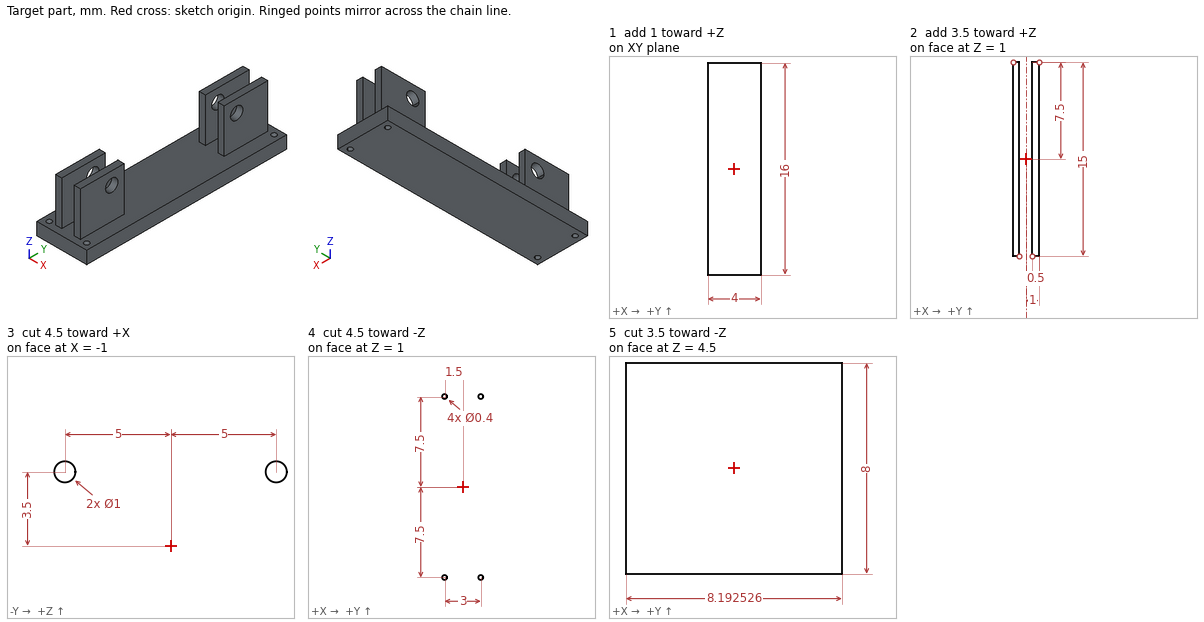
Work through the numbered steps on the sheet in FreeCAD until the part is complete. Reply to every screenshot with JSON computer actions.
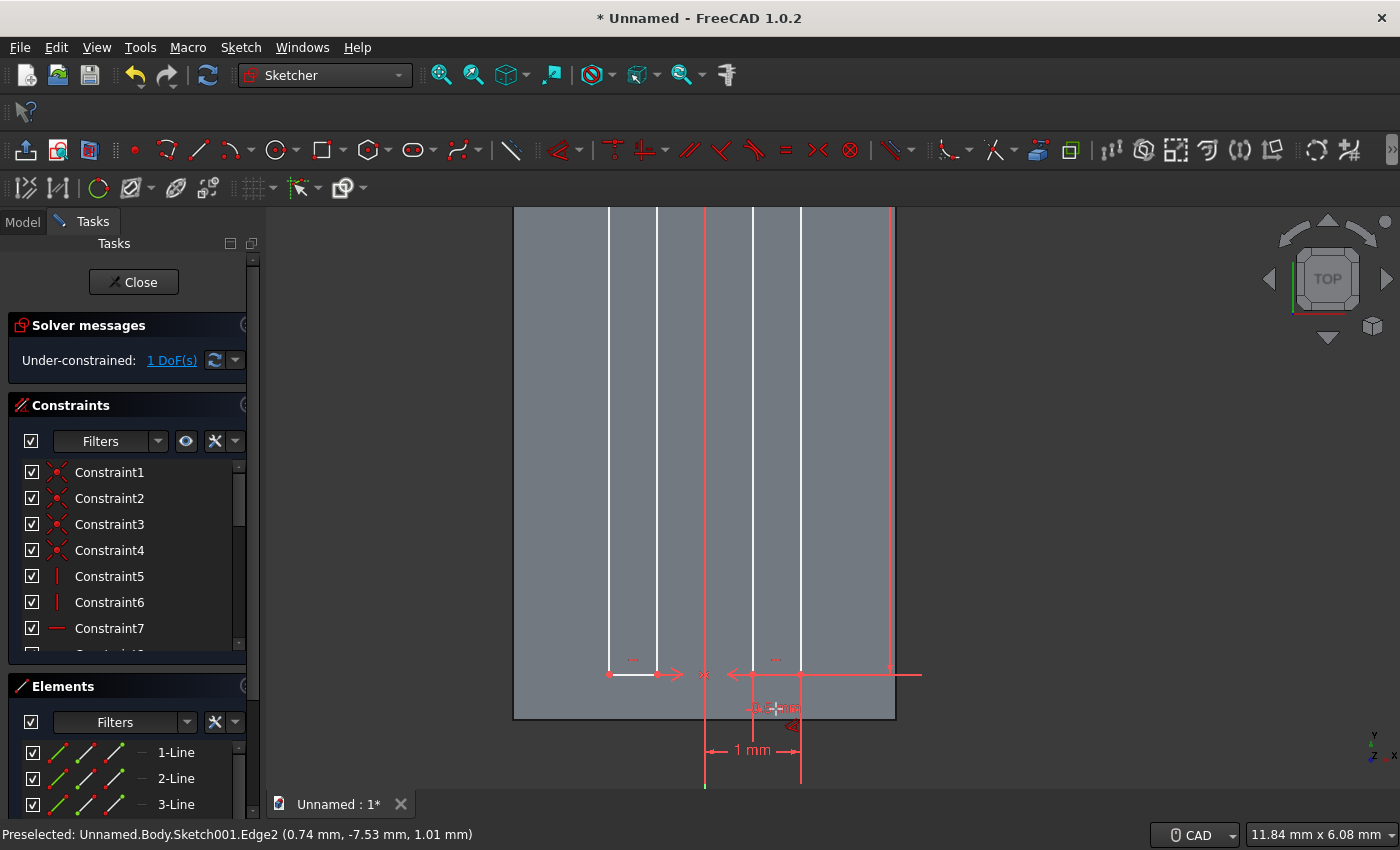
{"action": "scroll", "coordinate": [784, 676], "scroll_direction": "down", "scroll_amount": 7}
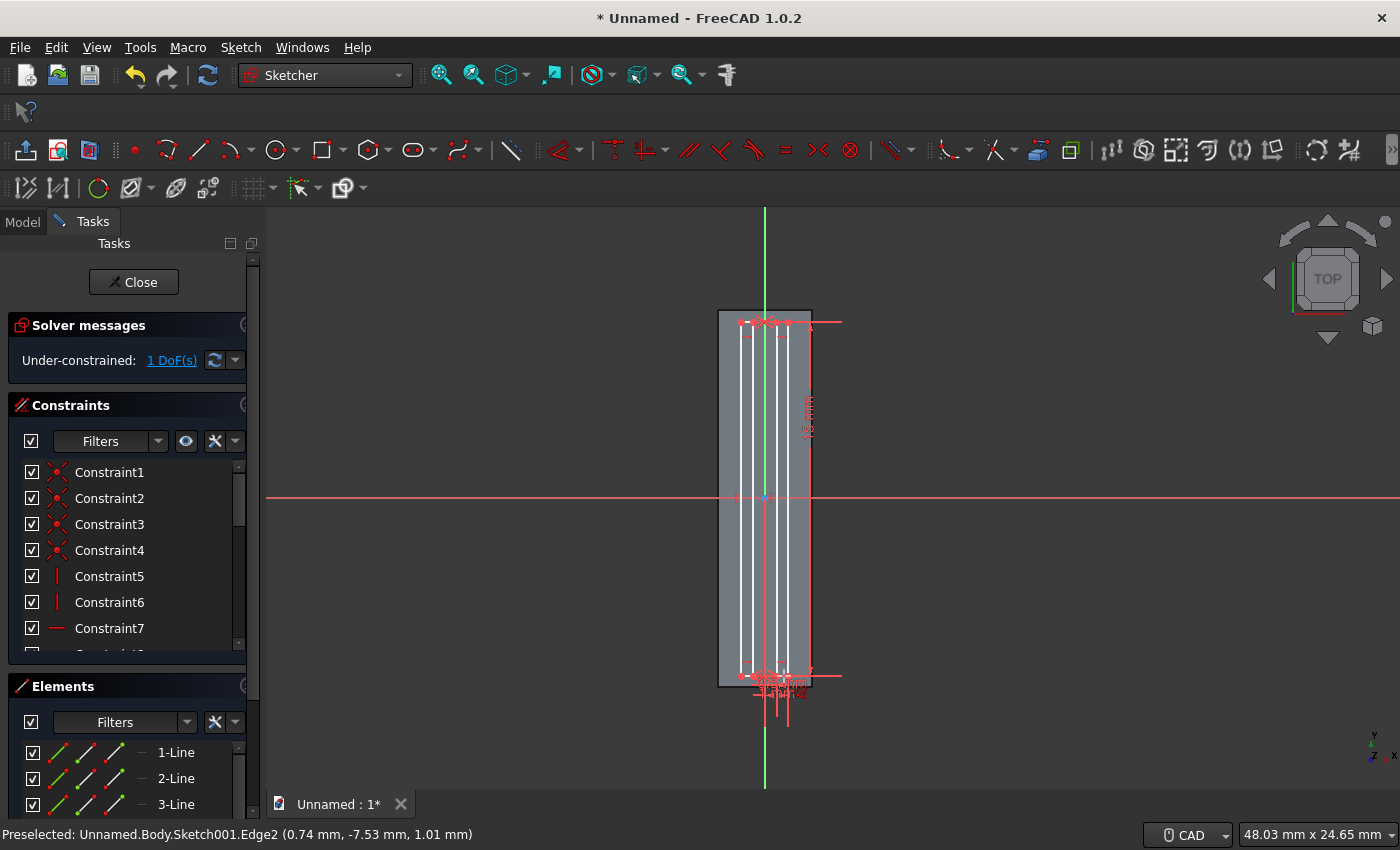
{"action": "left_click", "coordinate": [777, 322]}
{"action": "left_click", "coordinate": [811, 370]}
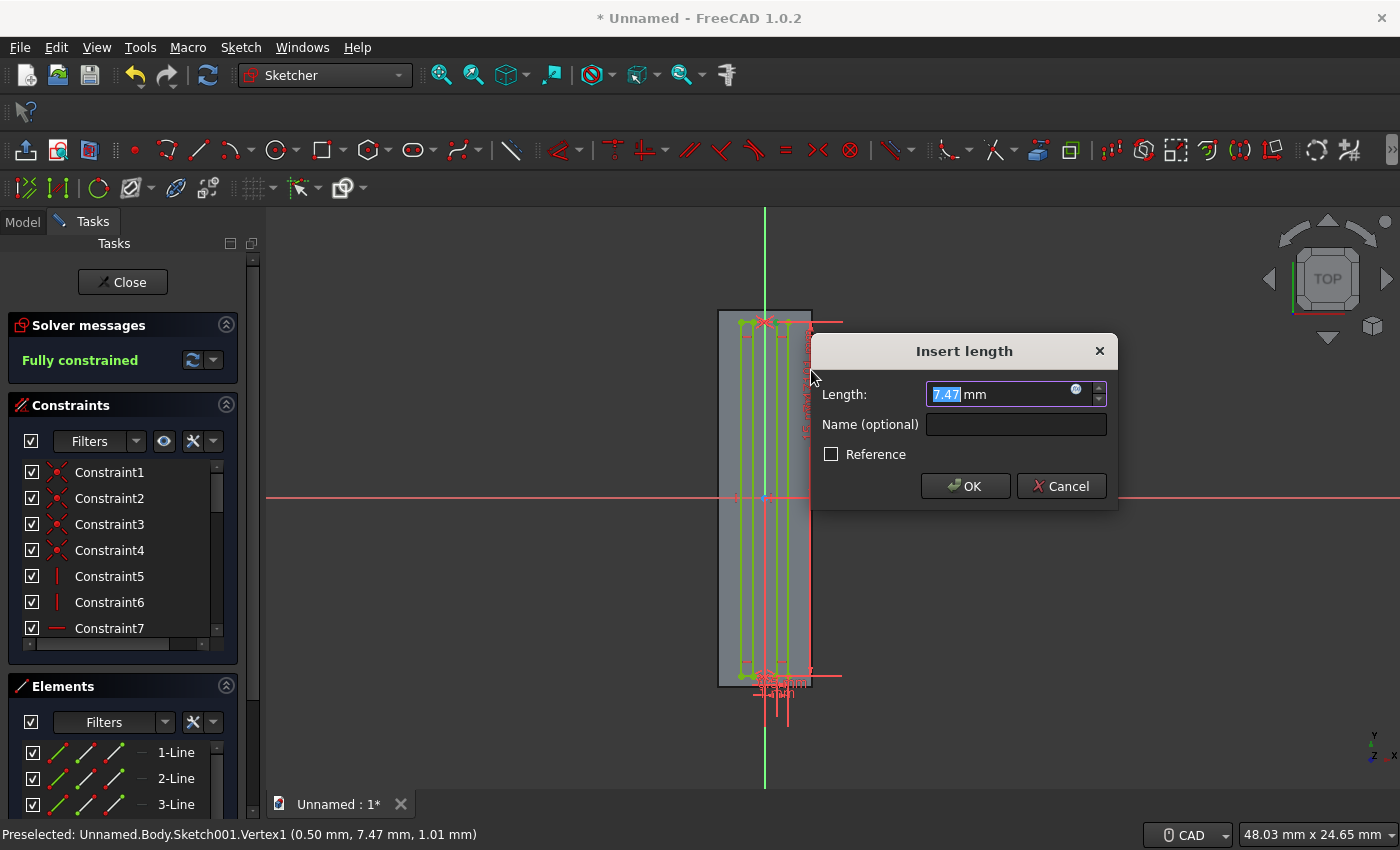
{"action": "type", "text": "7.5"}
{"action": "key", "text": "Return"}
{"action": "key", "text": "Escape"}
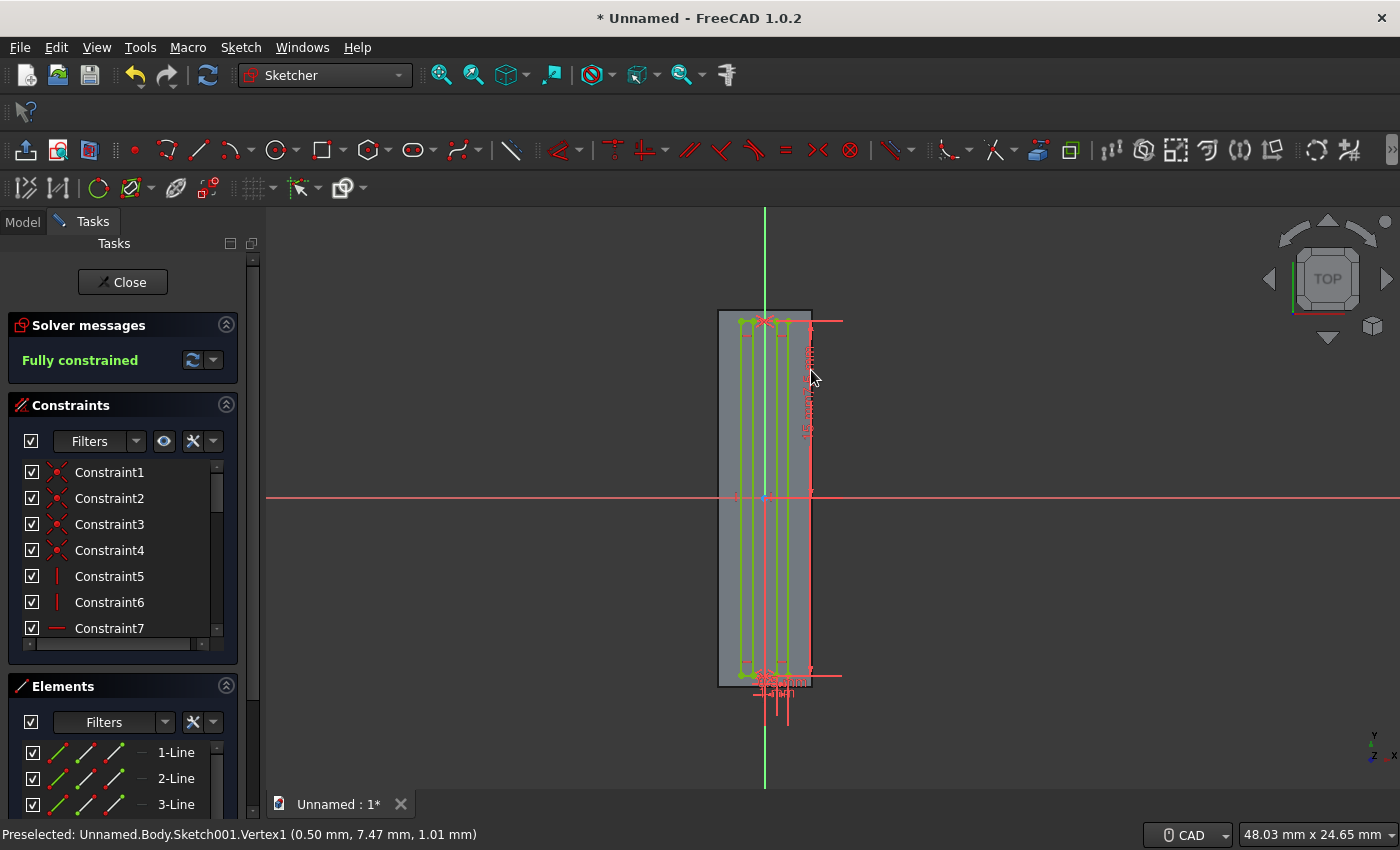
{"action": "left_click", "coordinate": [123, 282]}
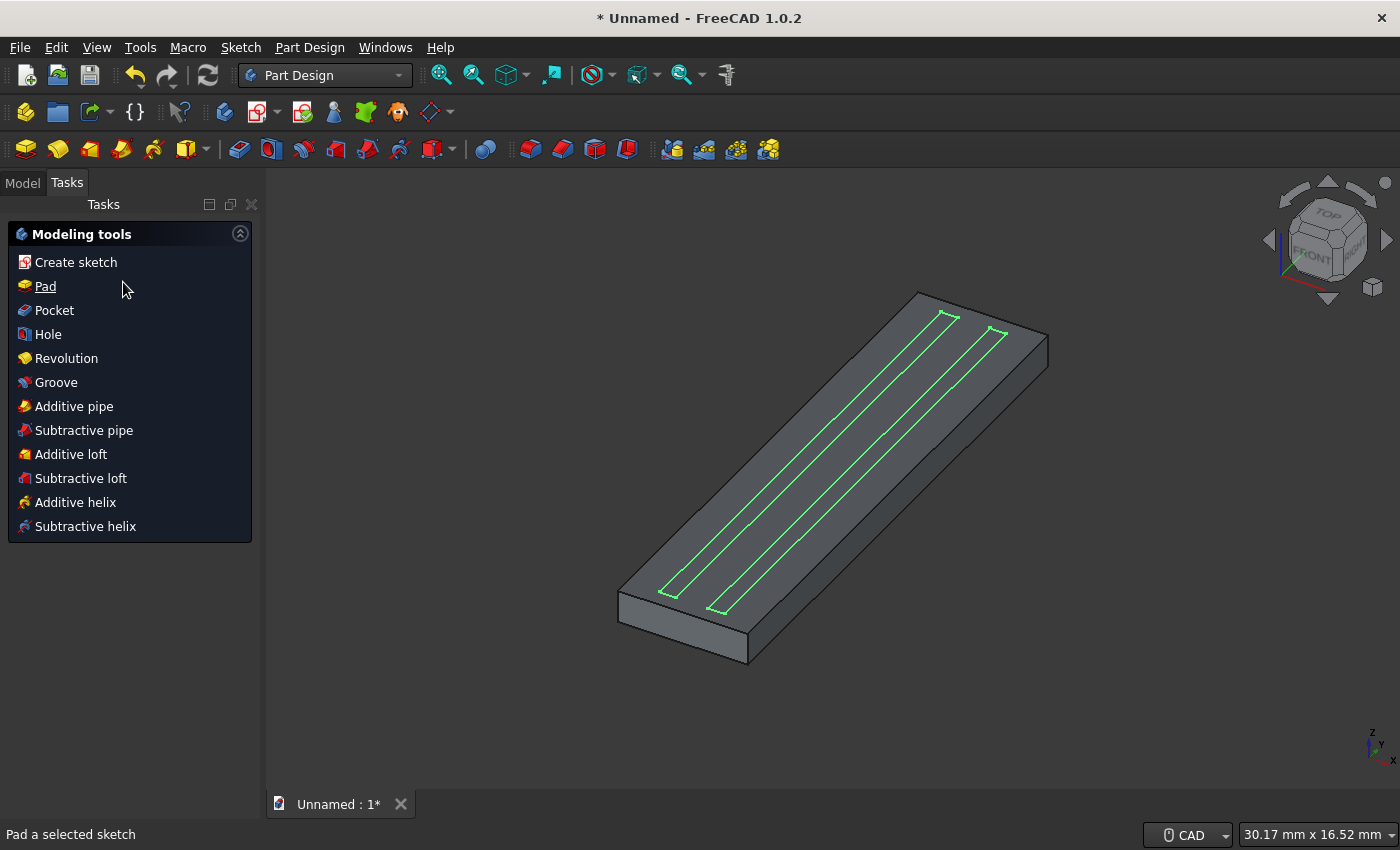
{"action": "left_click", "coordinate": [26, 150]}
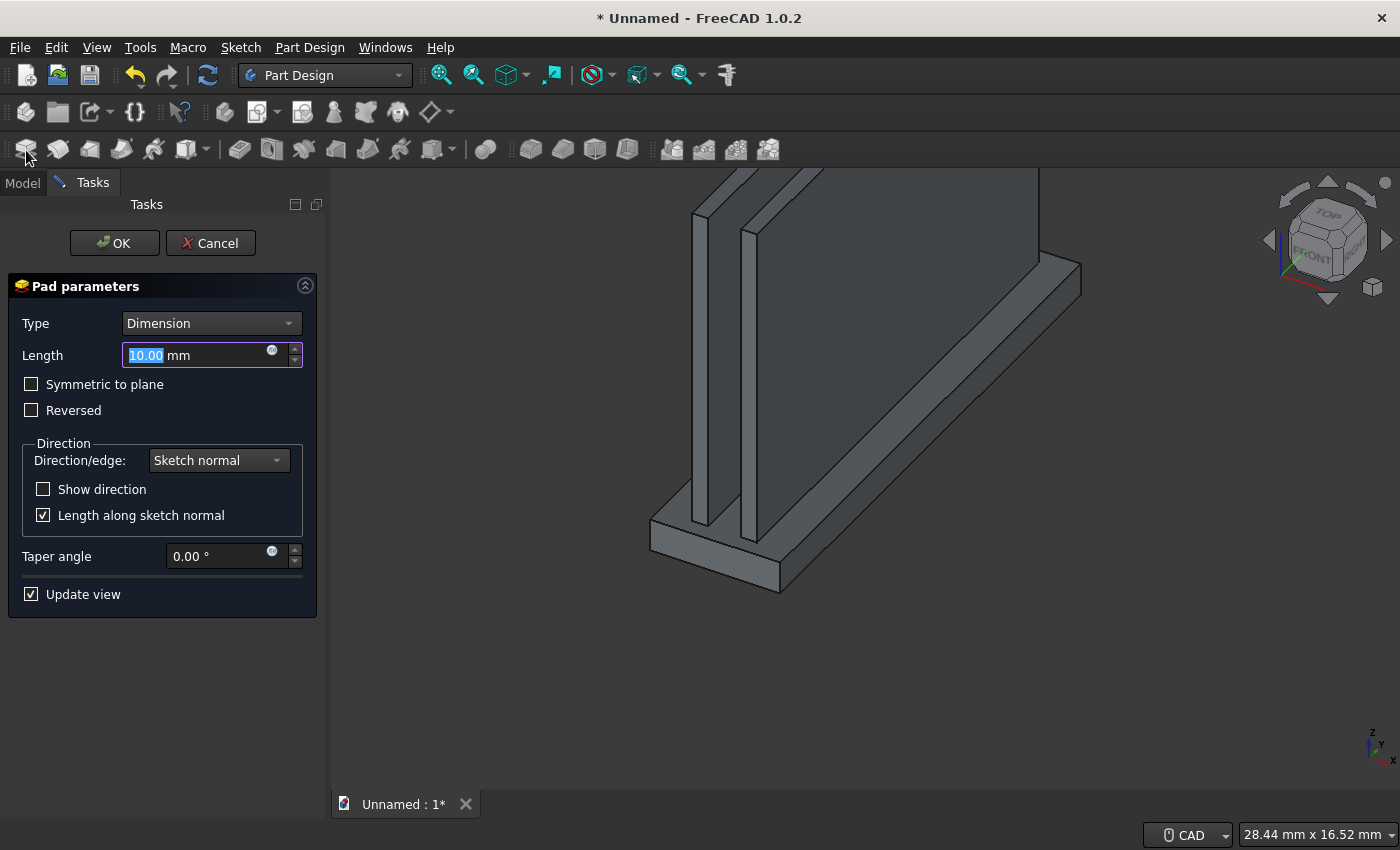
{"action": "type", "text": "3.5"}
{"action": "key", "text": "Tab"}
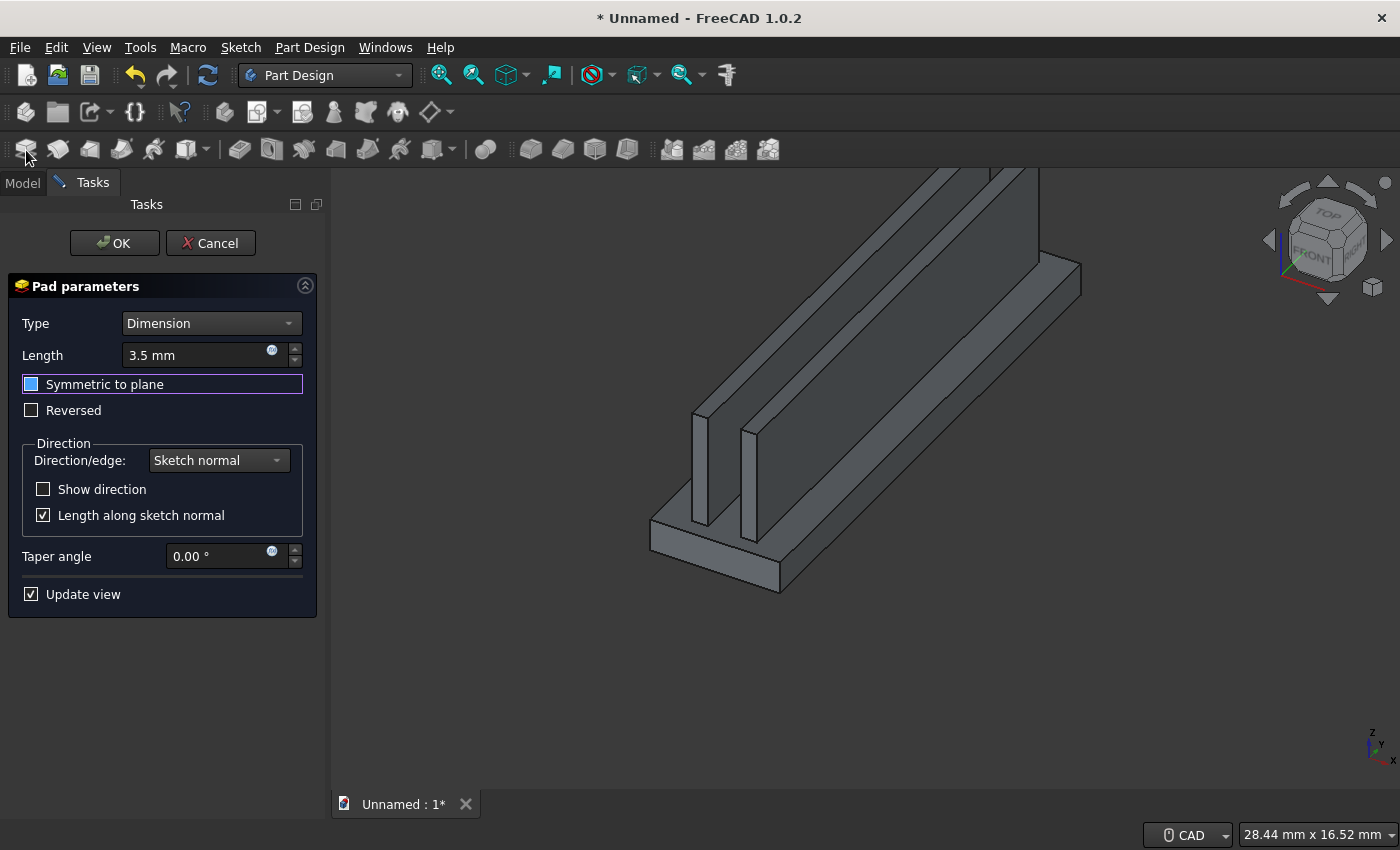
{"action": "left_click", "coordinate": [115, 243]}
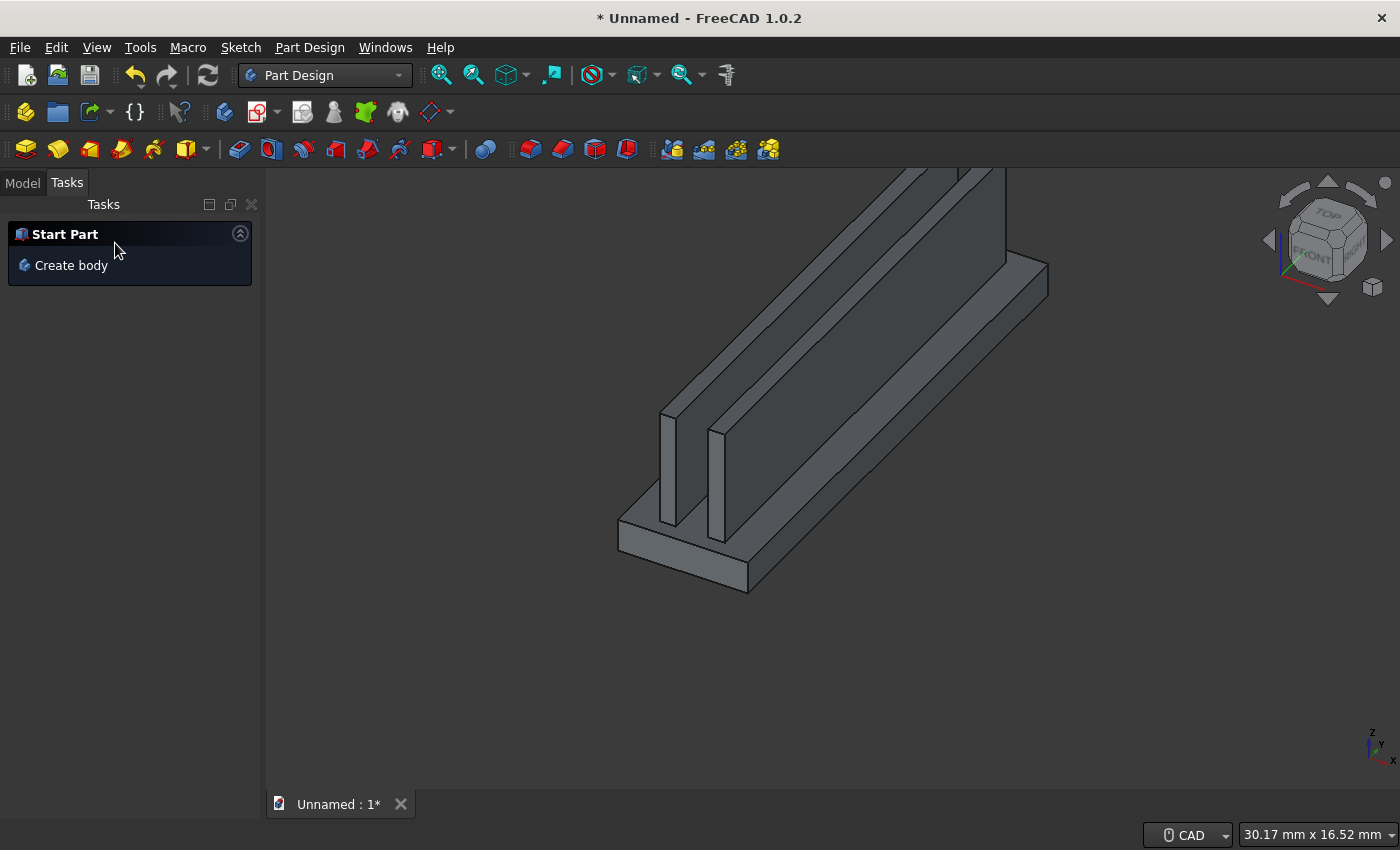
{"action": "key", "text": "v f"}